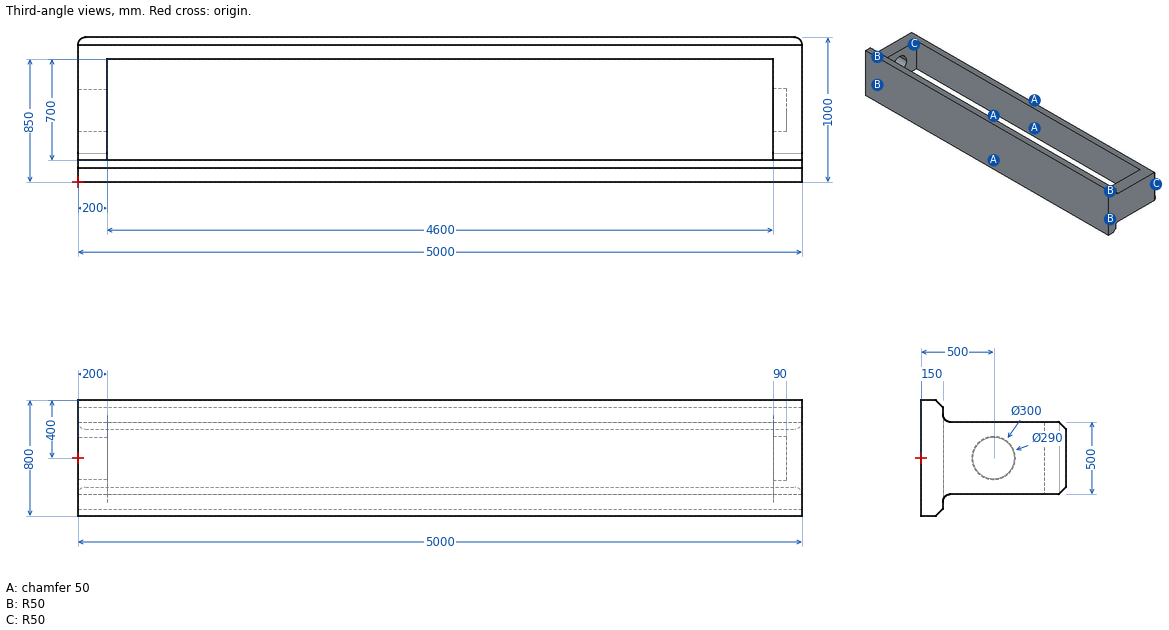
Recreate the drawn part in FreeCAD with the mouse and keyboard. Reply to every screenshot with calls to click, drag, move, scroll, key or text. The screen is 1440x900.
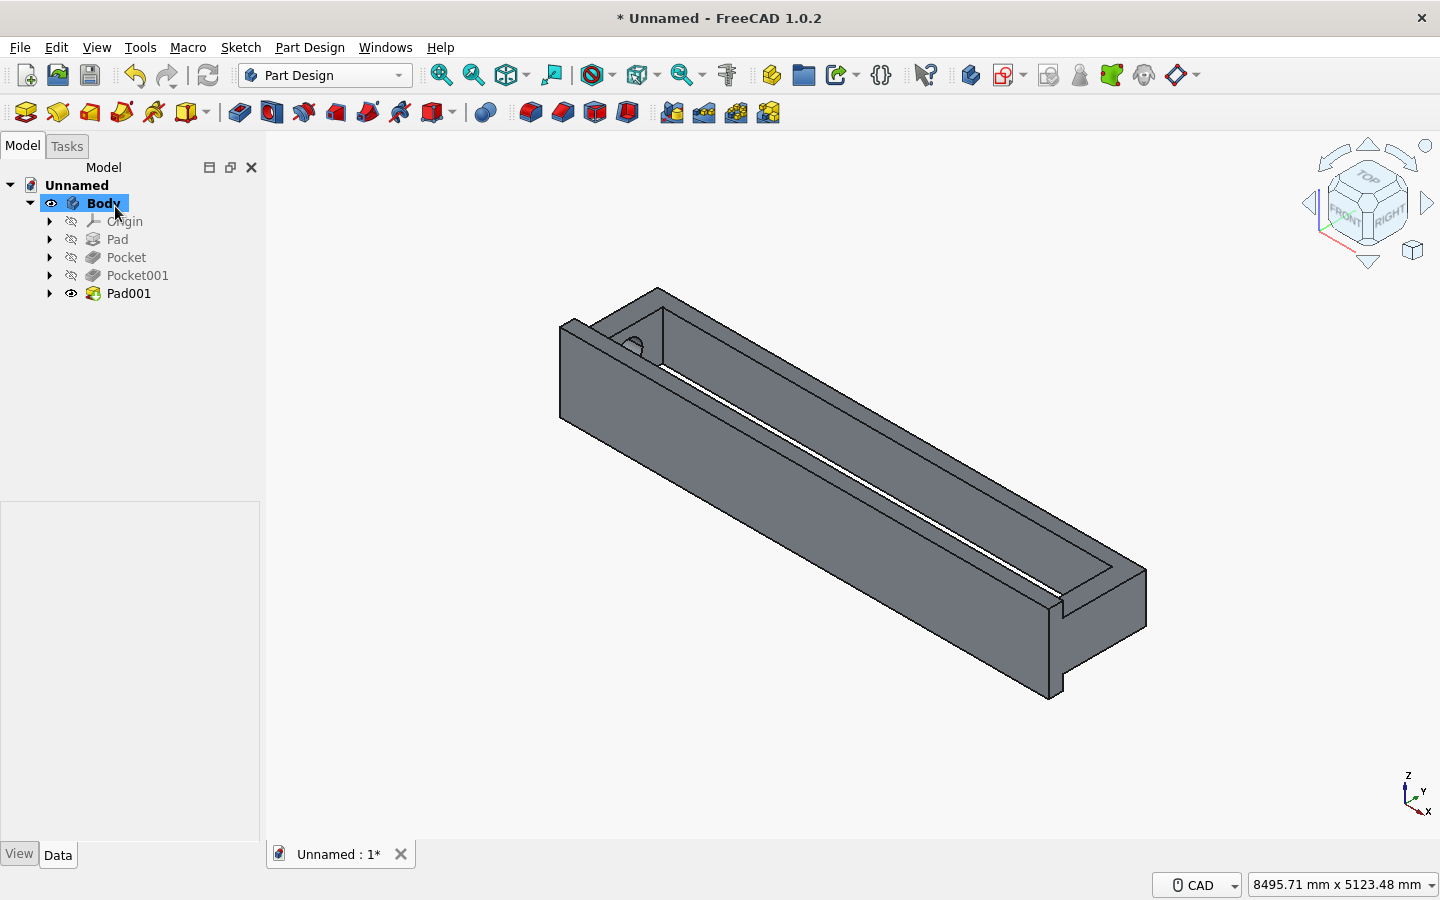
key(2)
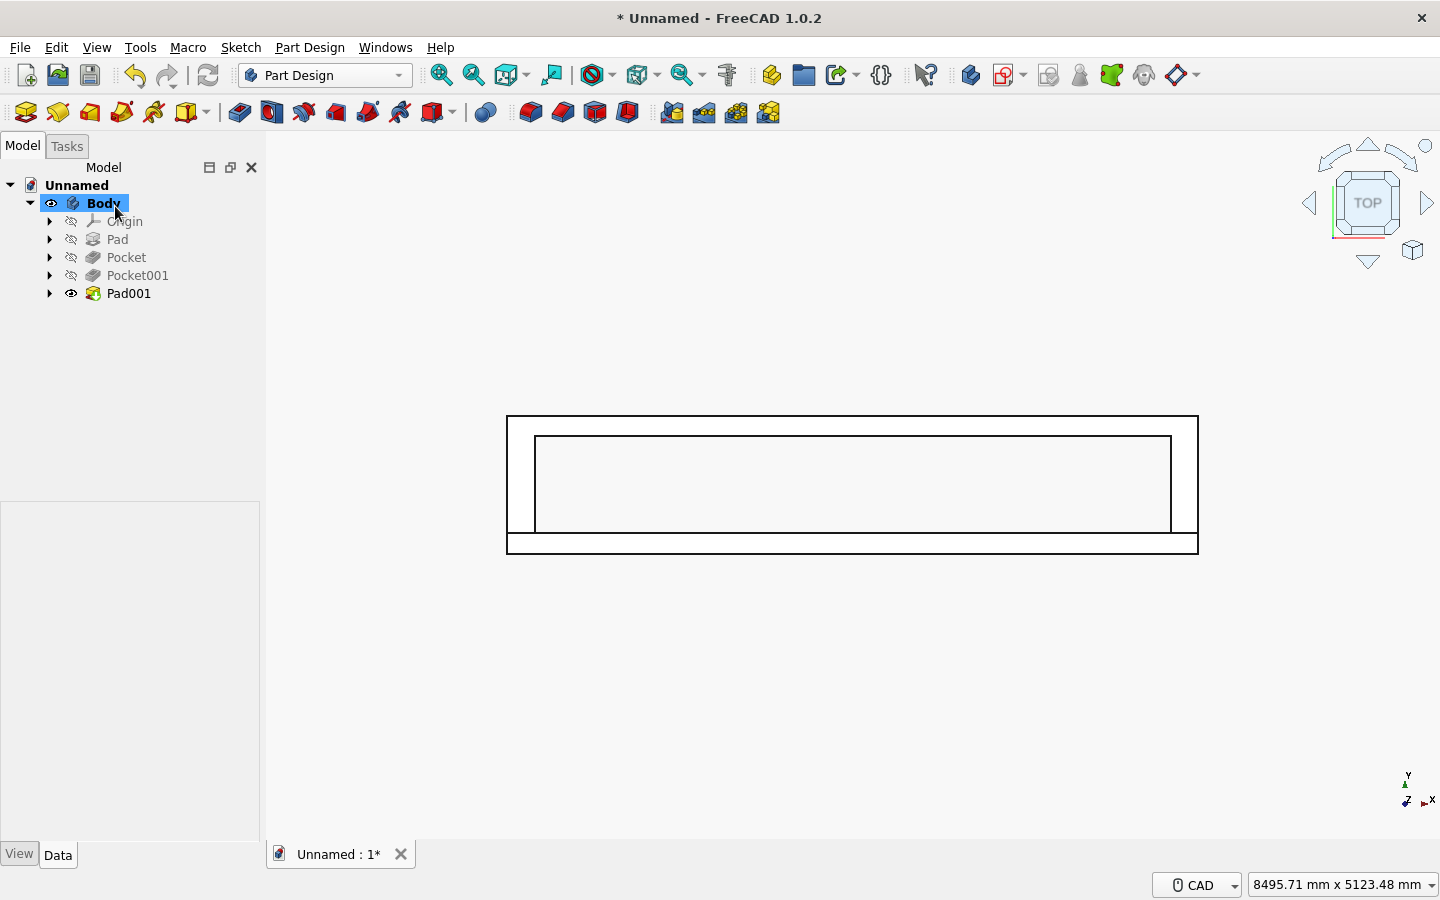
click(853, 532)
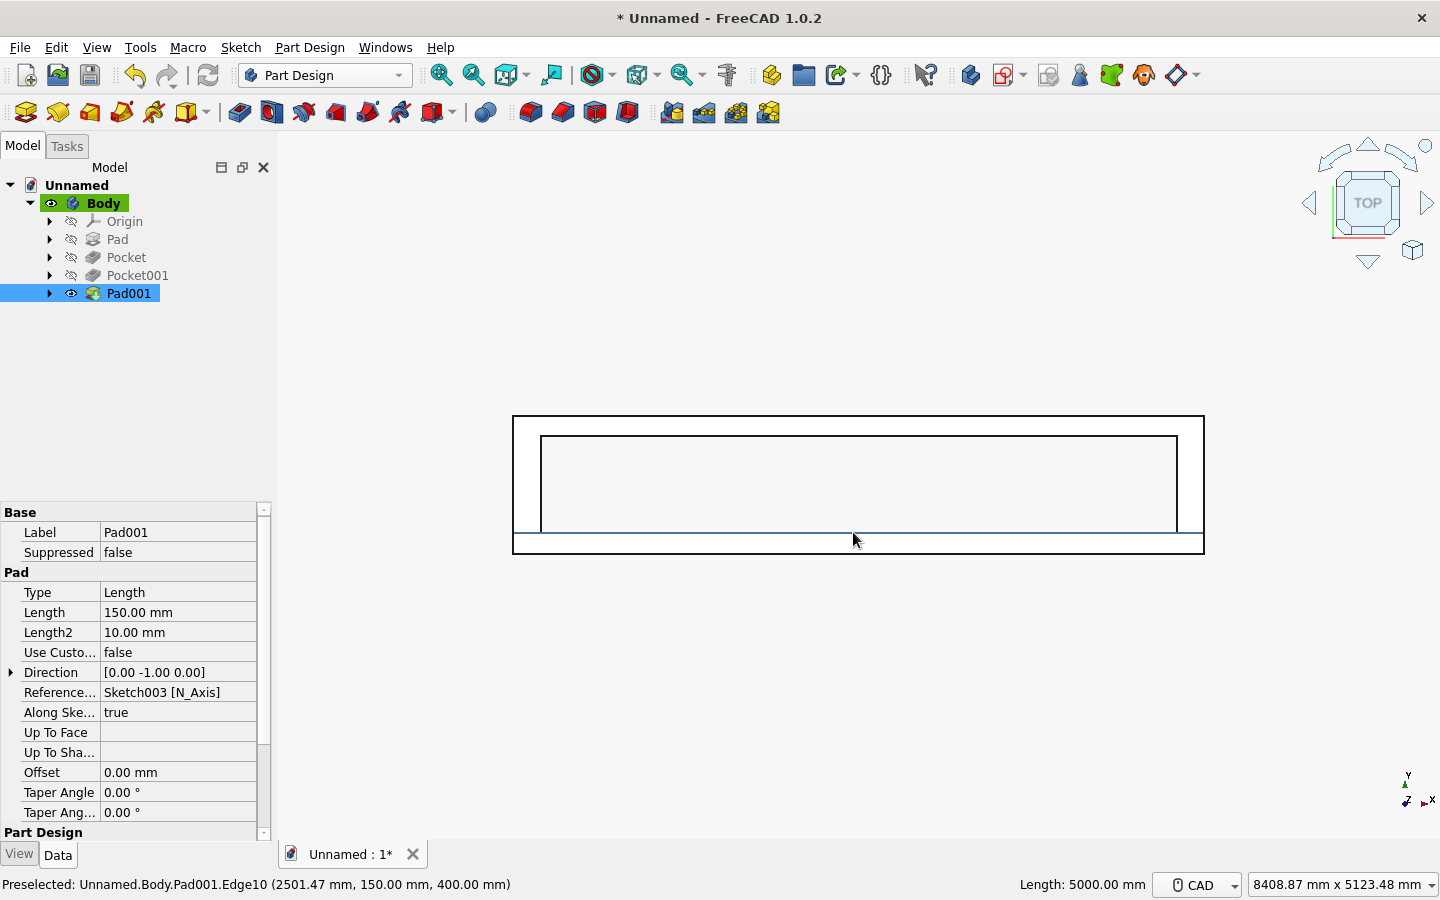
click(859, 415, ctrl)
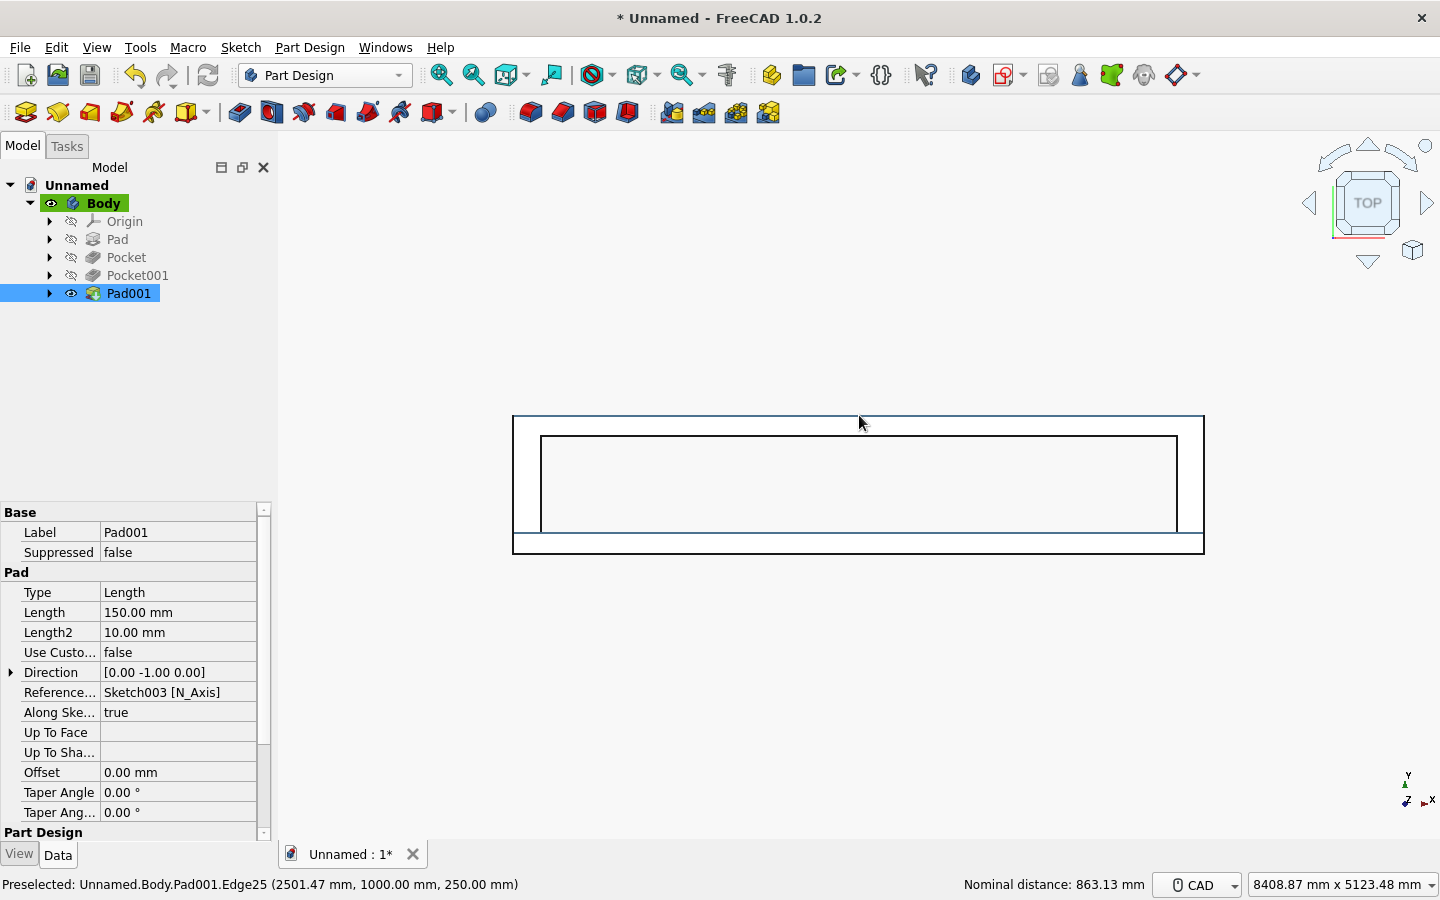
key(1)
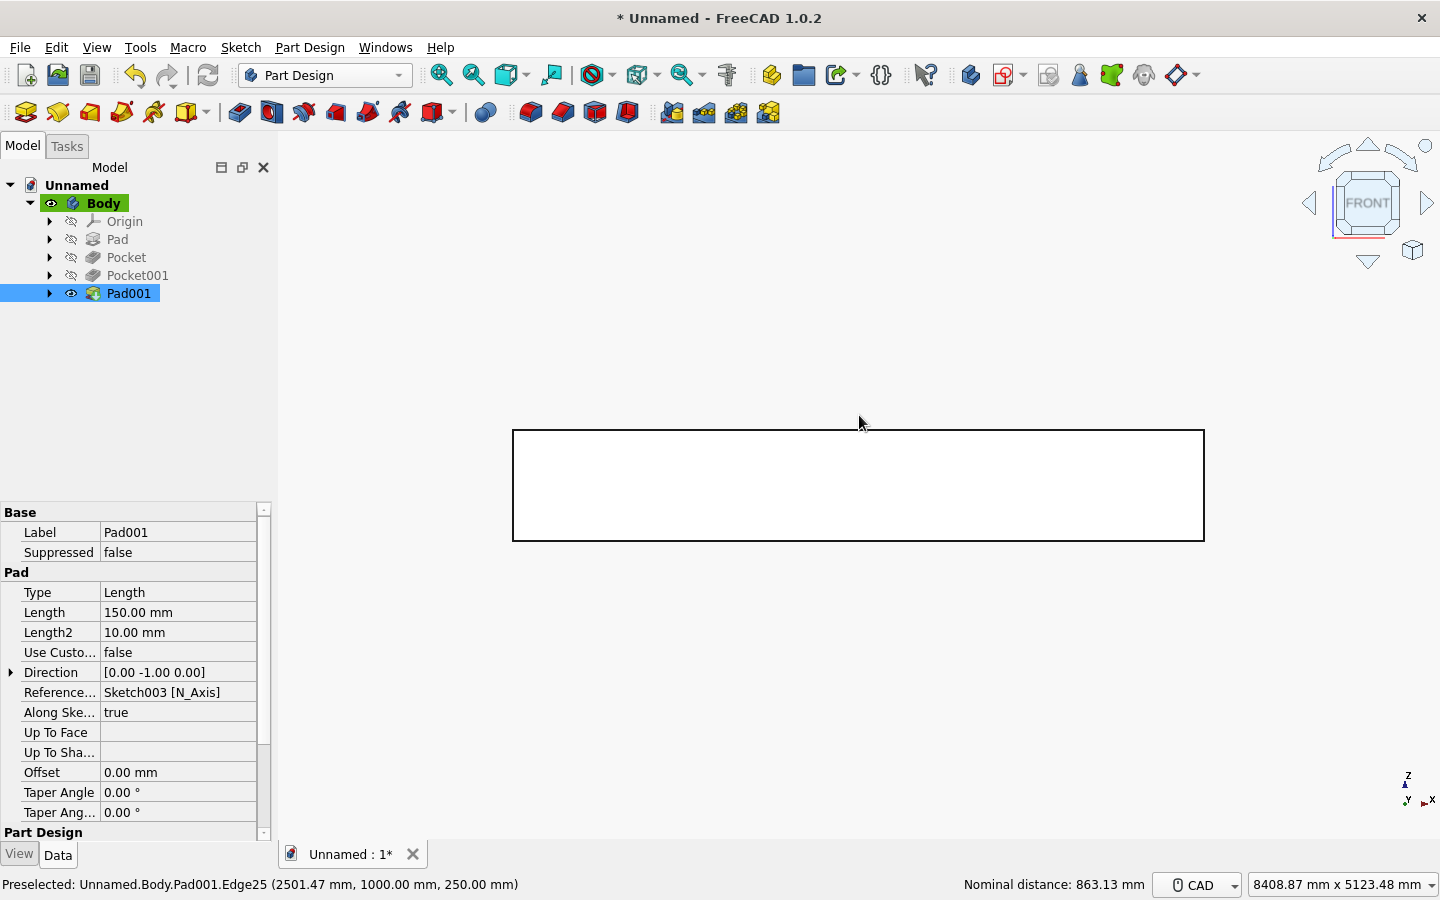
key(3)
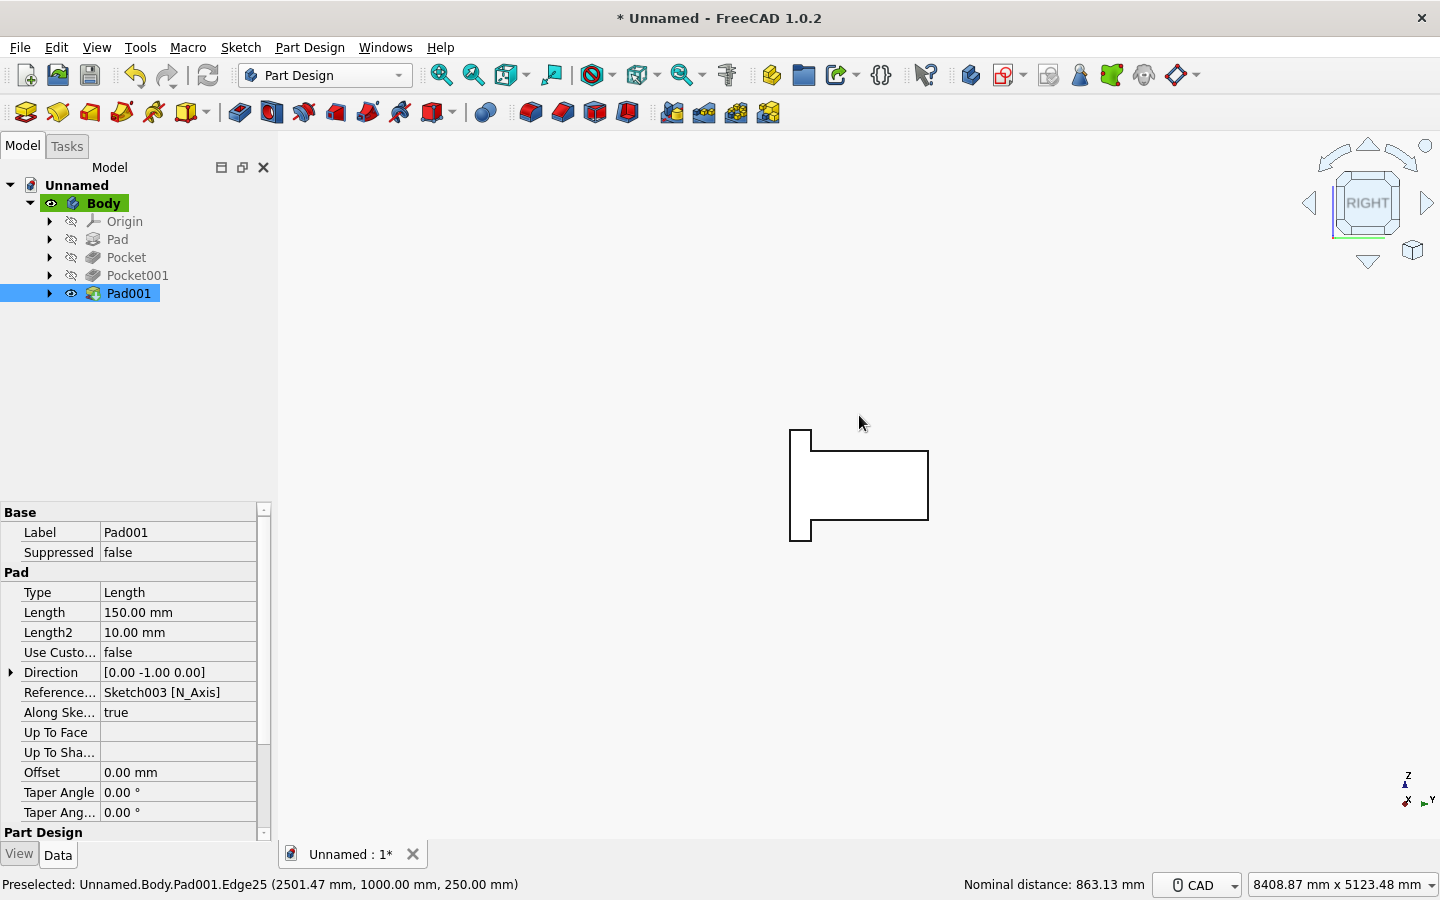
key(v)
key(f)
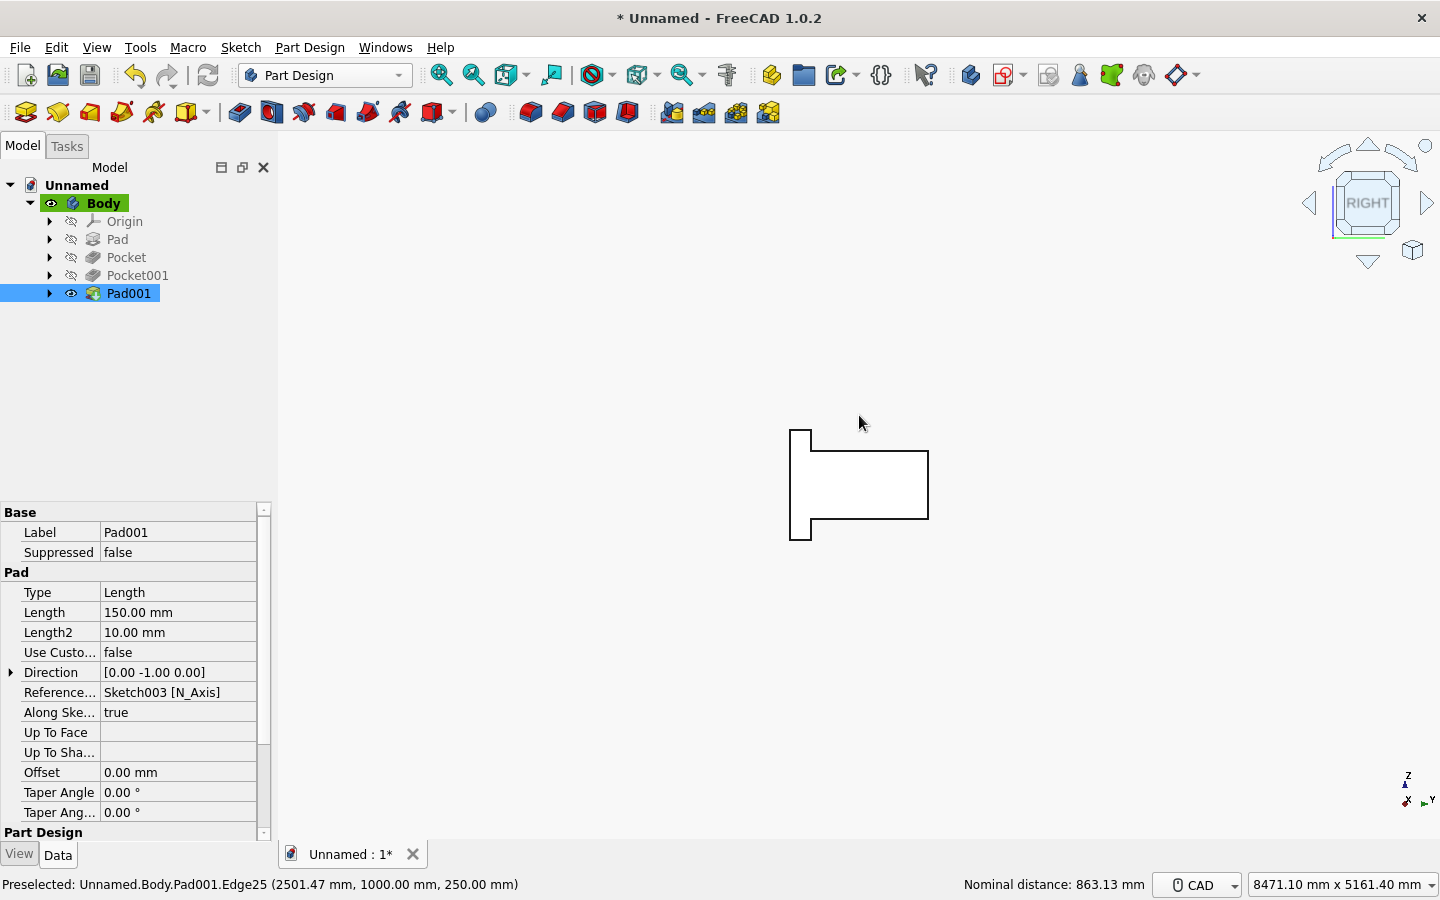
key(5)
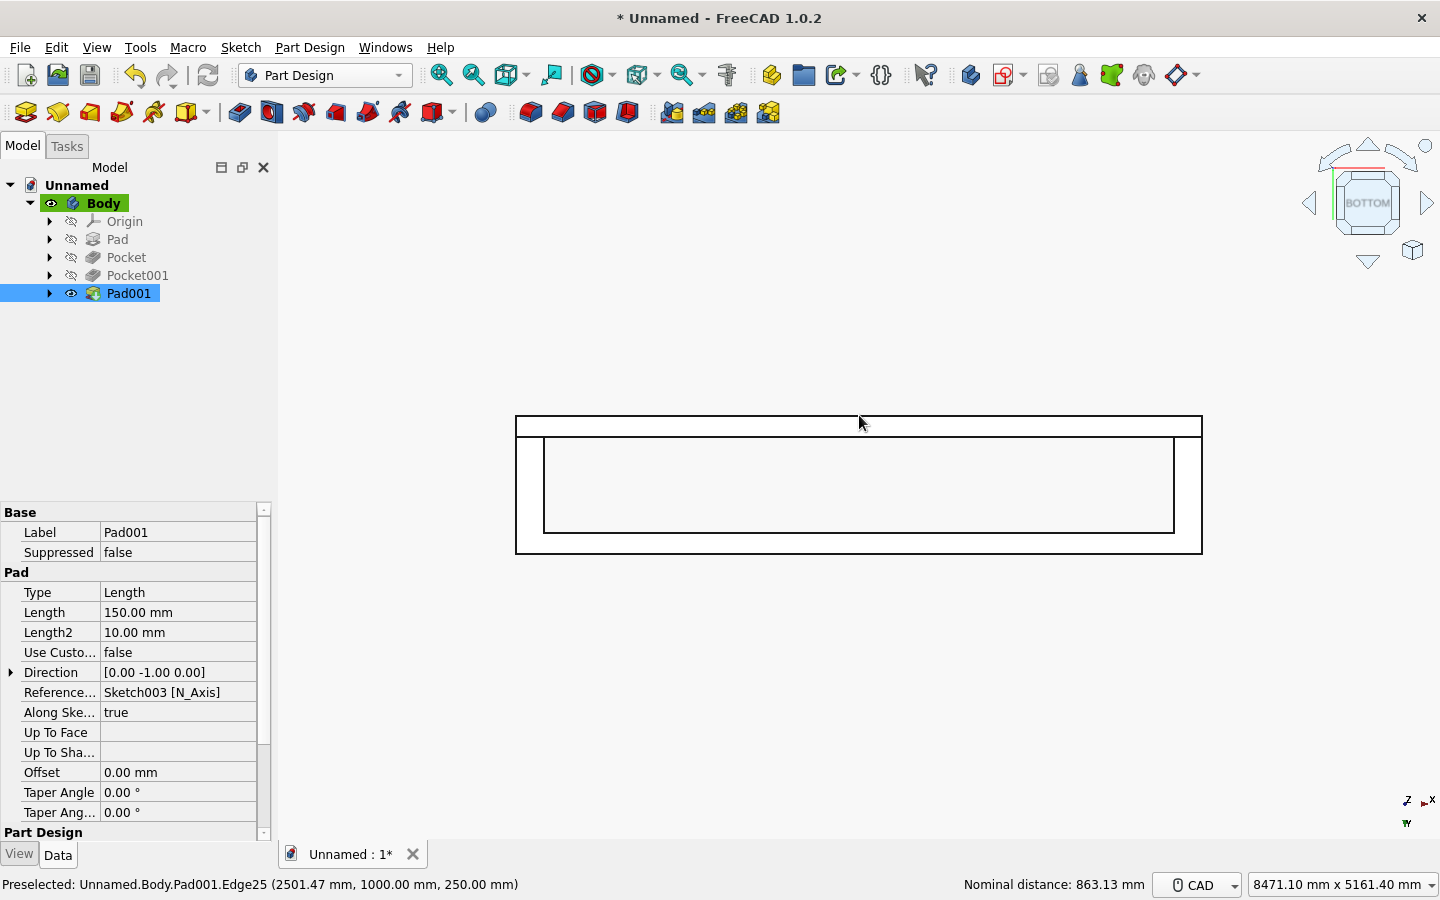
click(859, 436, ctrl)